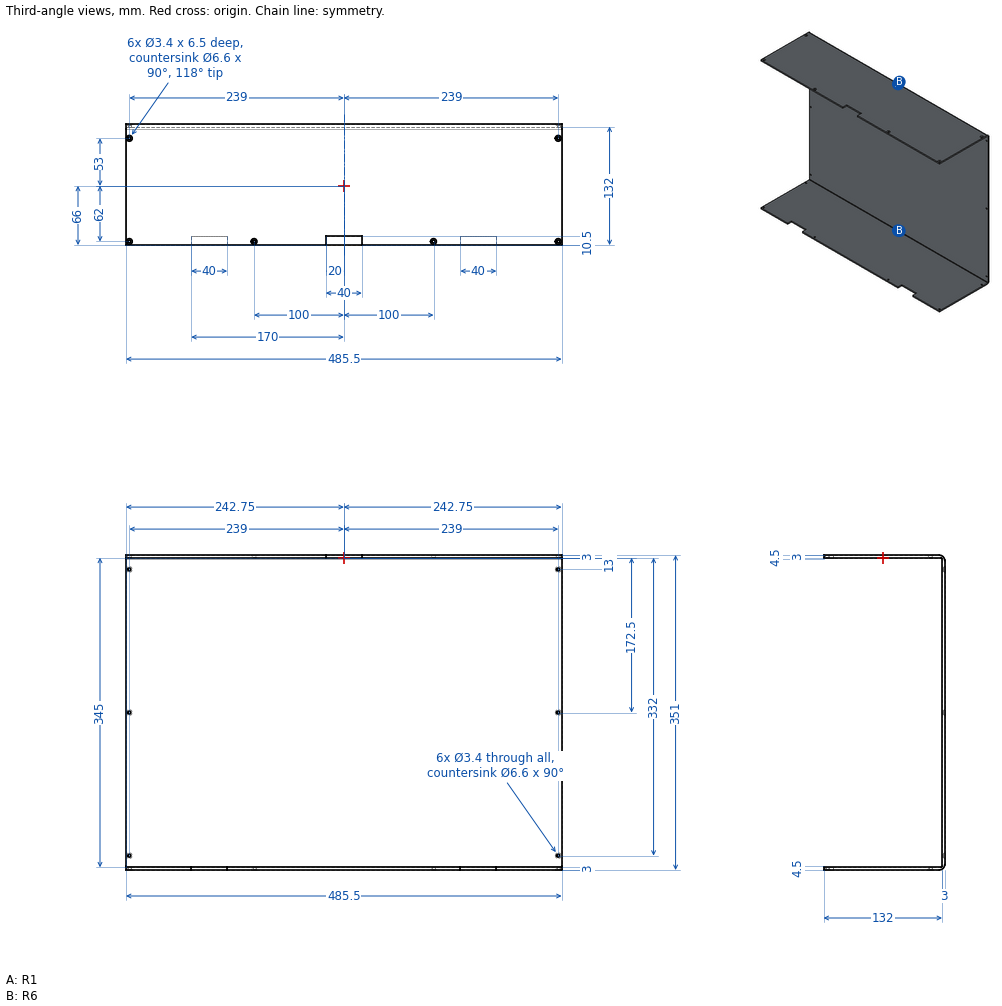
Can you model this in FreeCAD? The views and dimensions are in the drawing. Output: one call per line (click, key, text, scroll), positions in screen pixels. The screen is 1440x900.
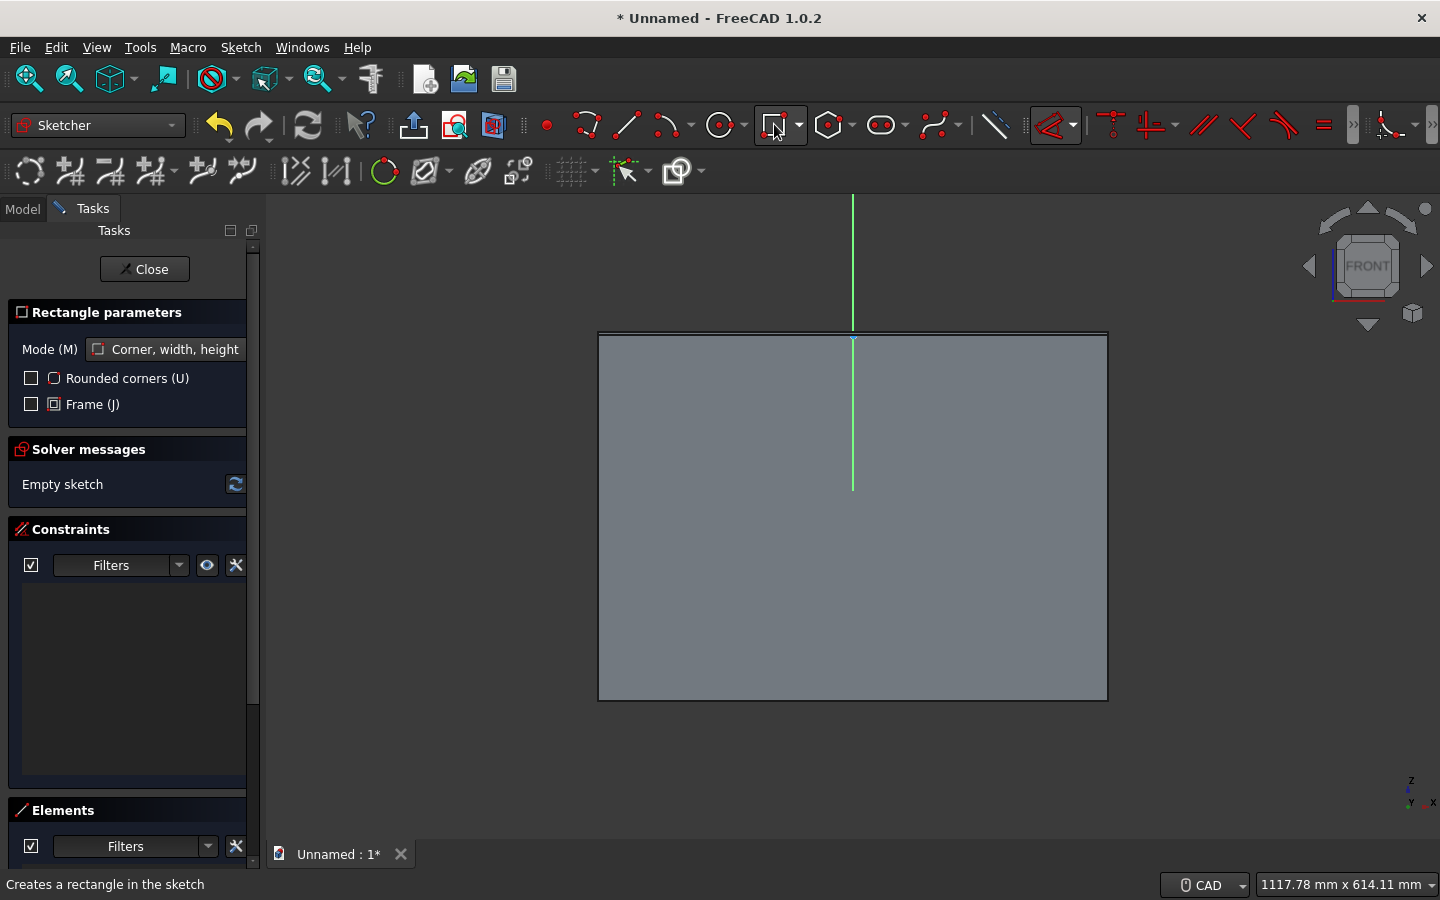
scroll(598, 698, up, 9)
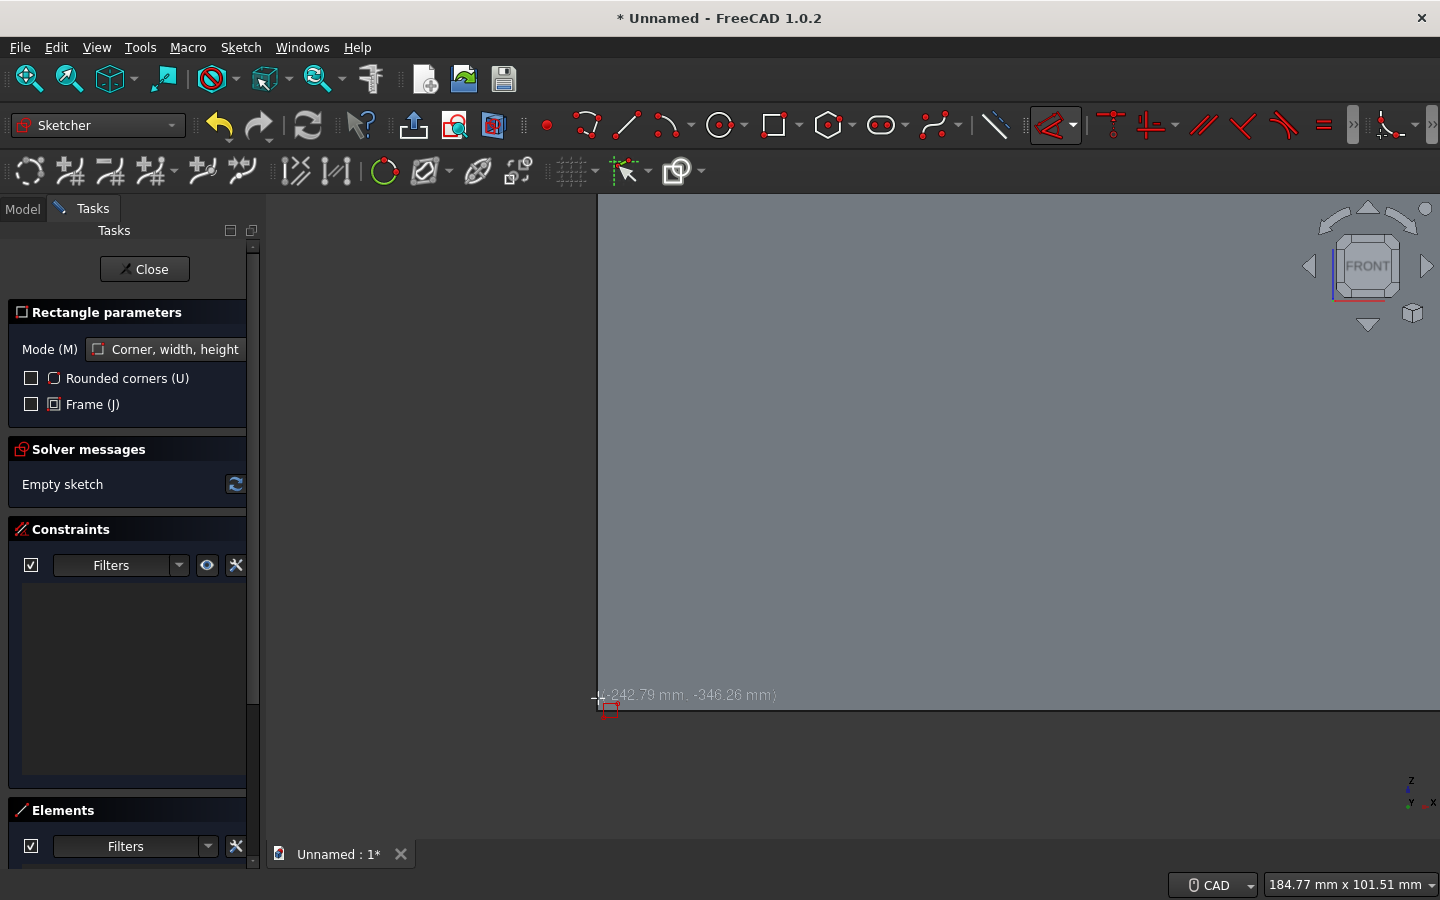
scroll(442, 747, down, 8)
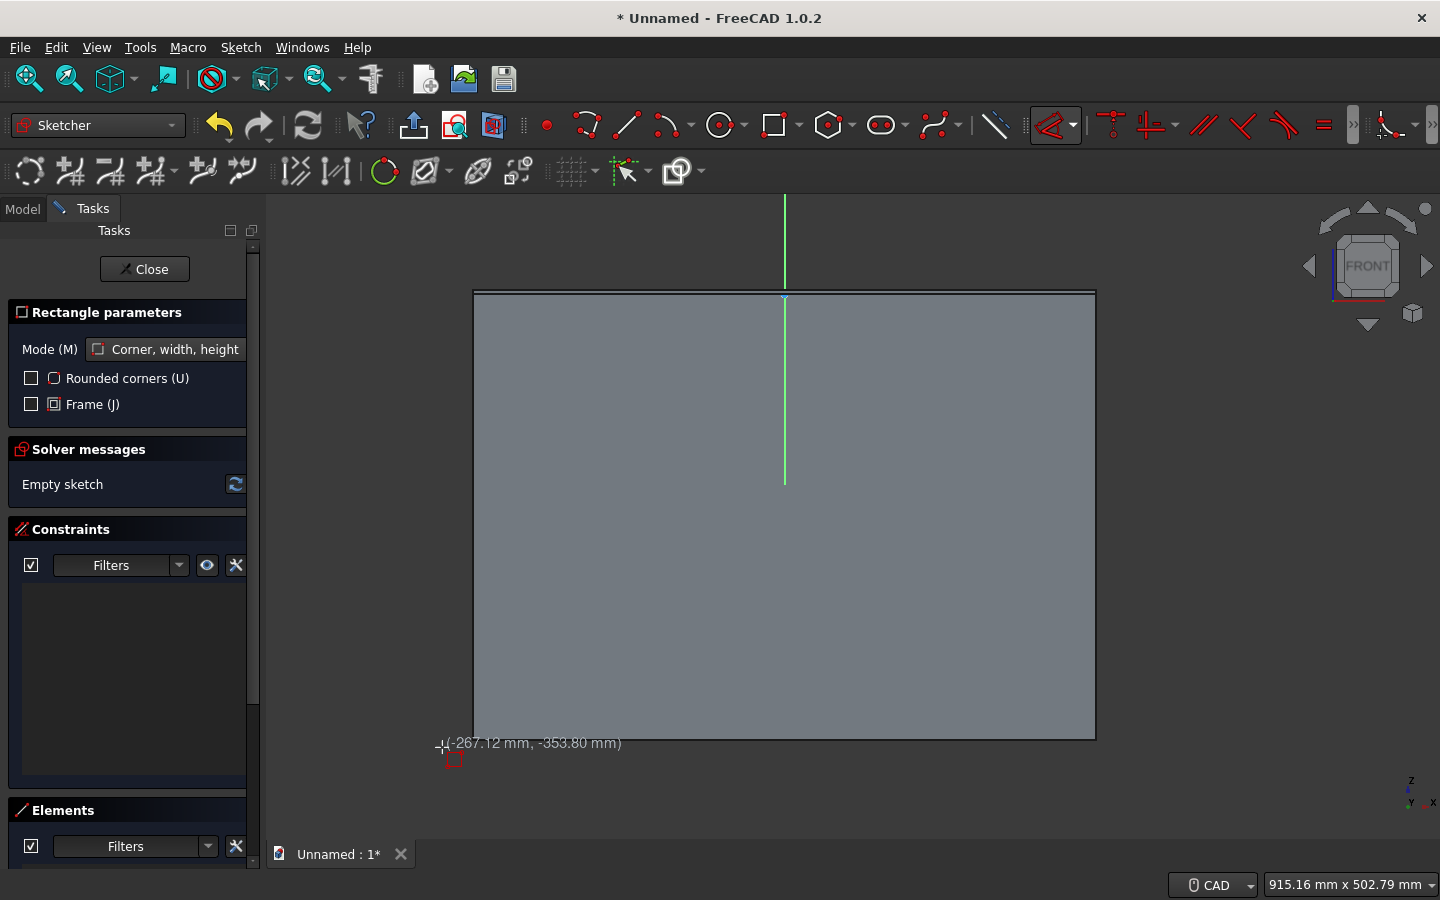
click(473, 737)
move(1096, 740)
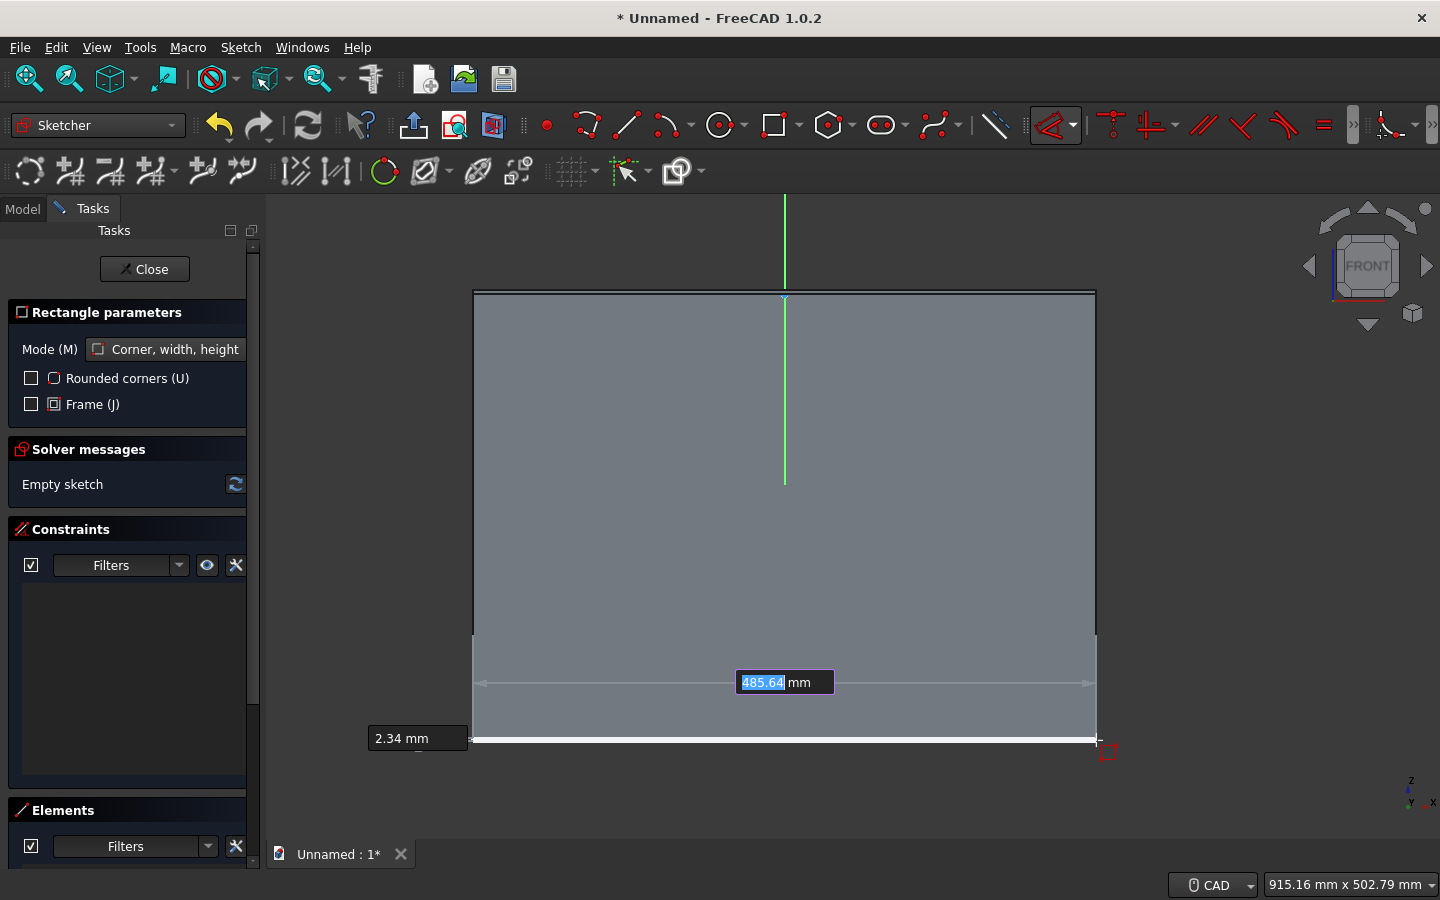
text(485.5)
key(Tab)
text(3)
key(Return)
key(Escape)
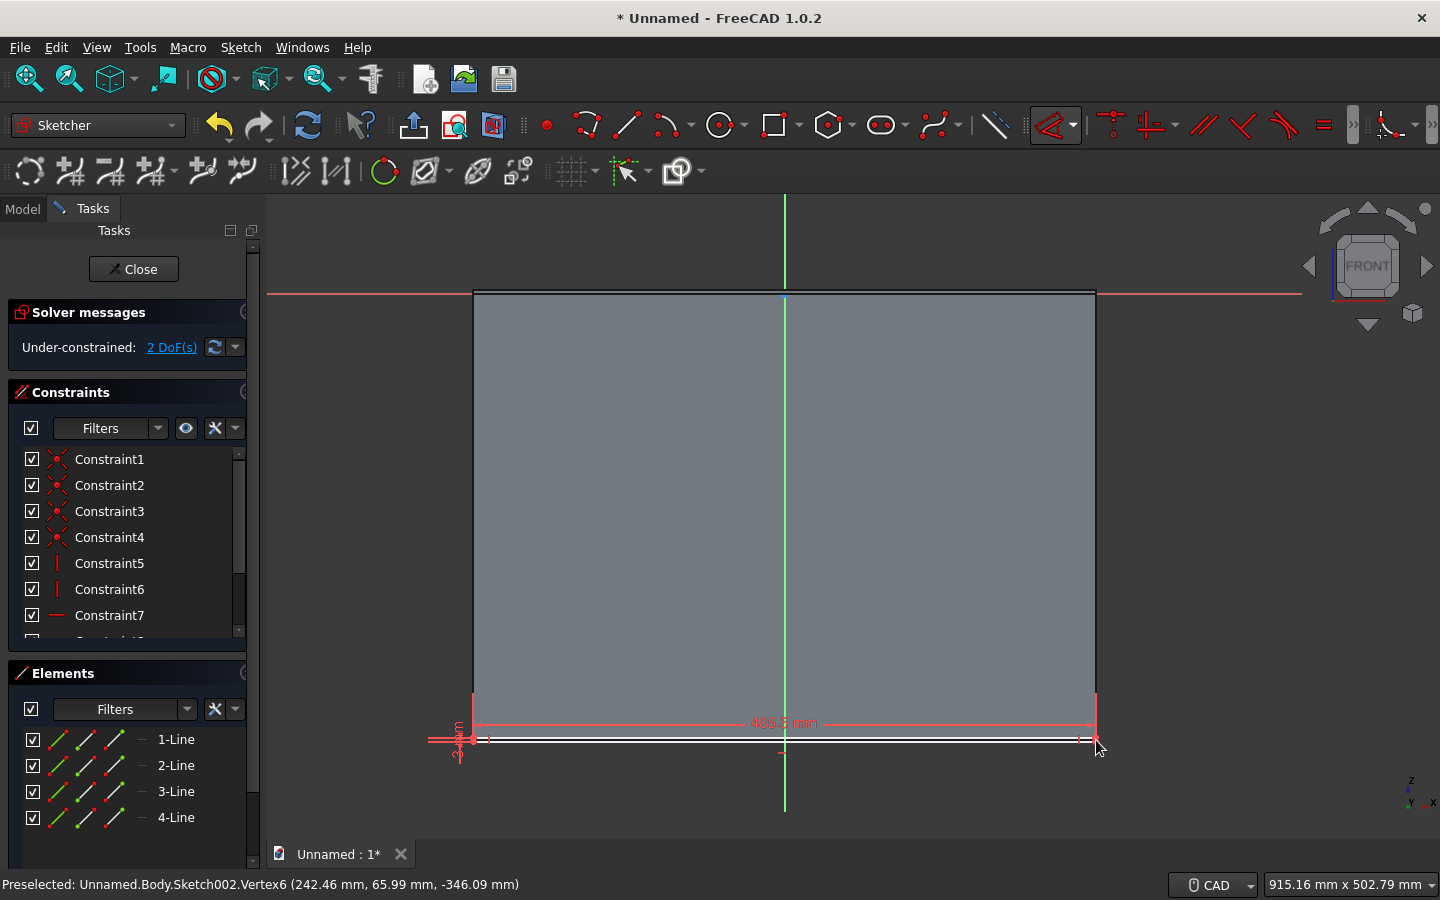
scroll(473, 738, up, 6)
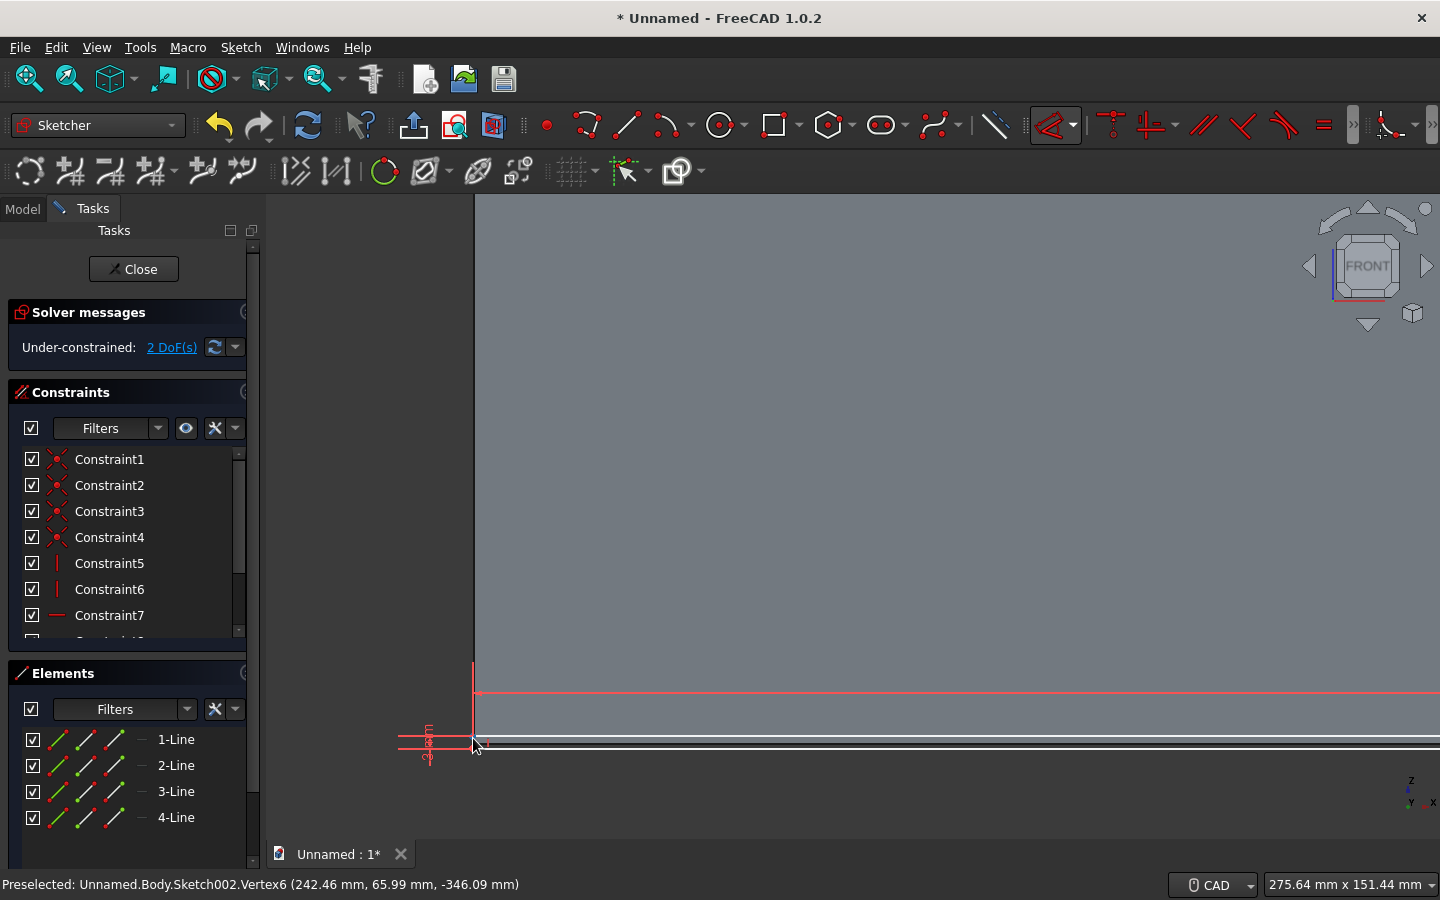
click(473, 736)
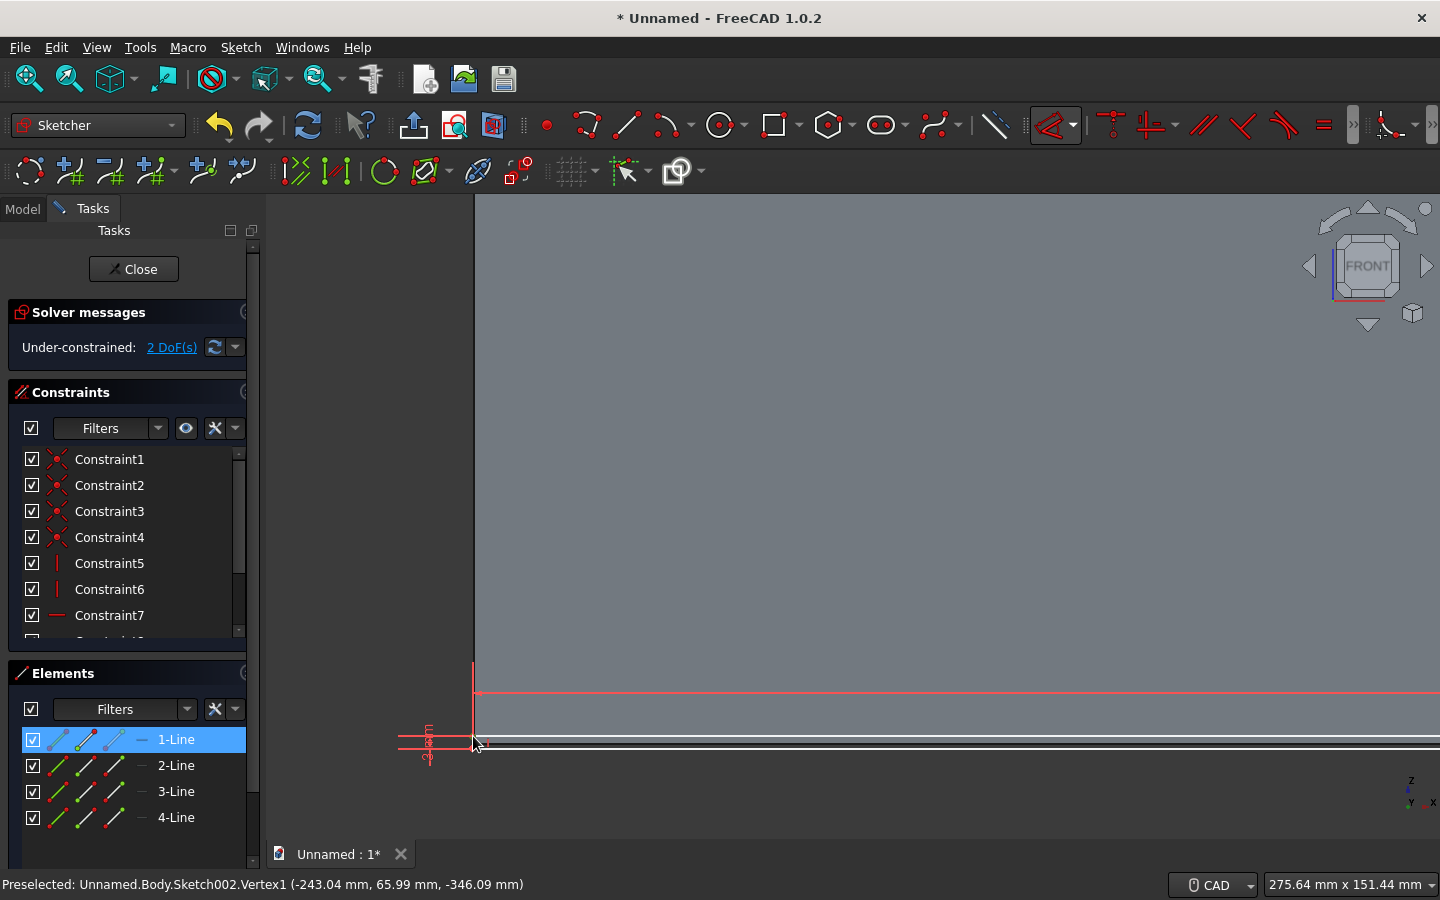
click(1076, 126)